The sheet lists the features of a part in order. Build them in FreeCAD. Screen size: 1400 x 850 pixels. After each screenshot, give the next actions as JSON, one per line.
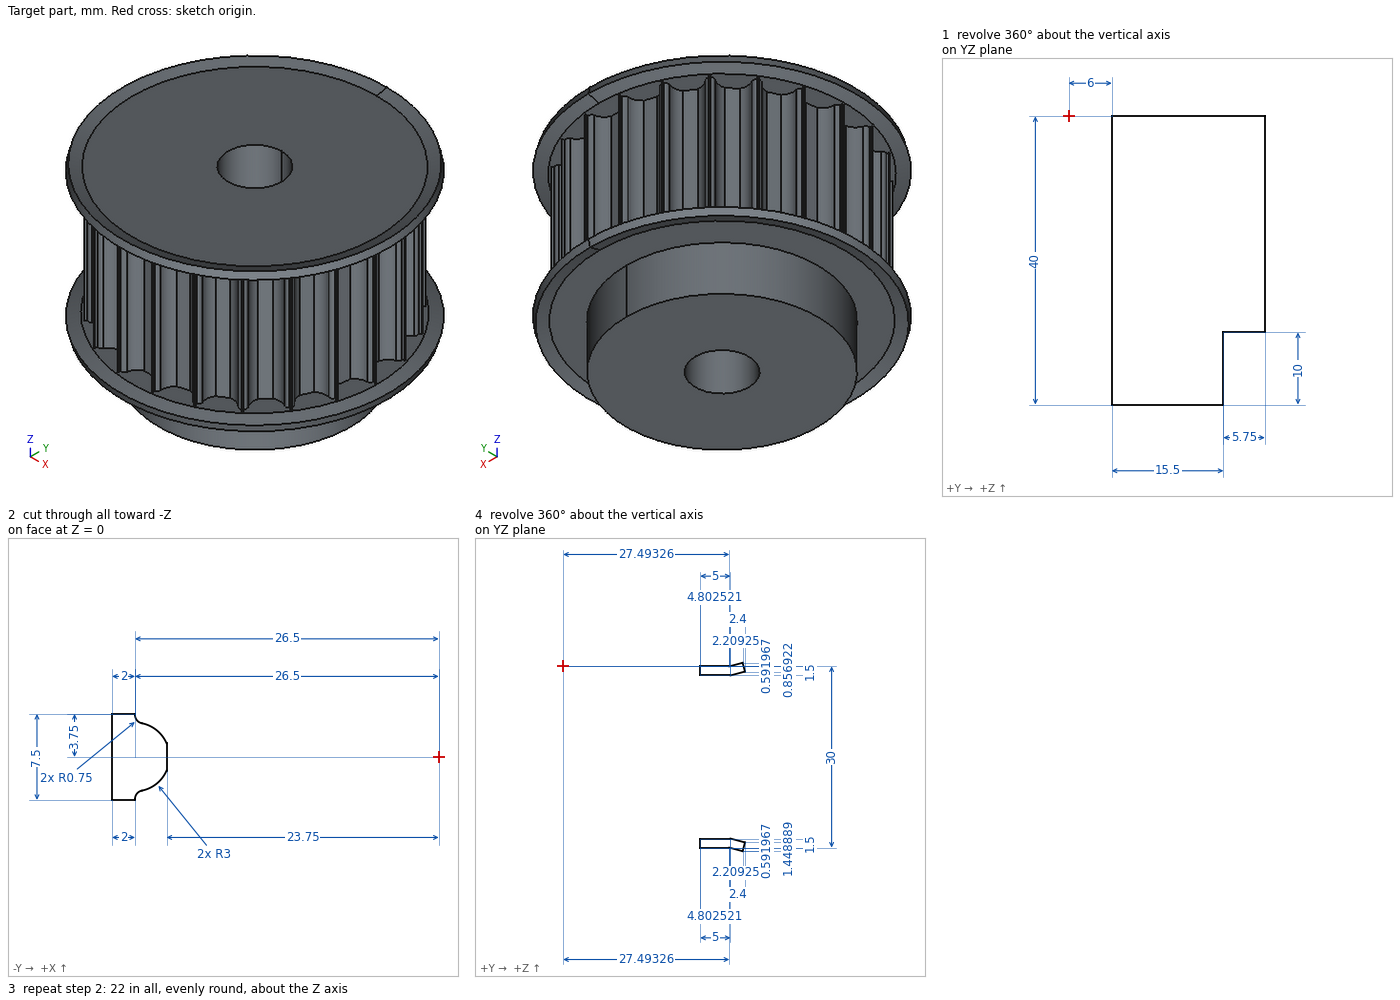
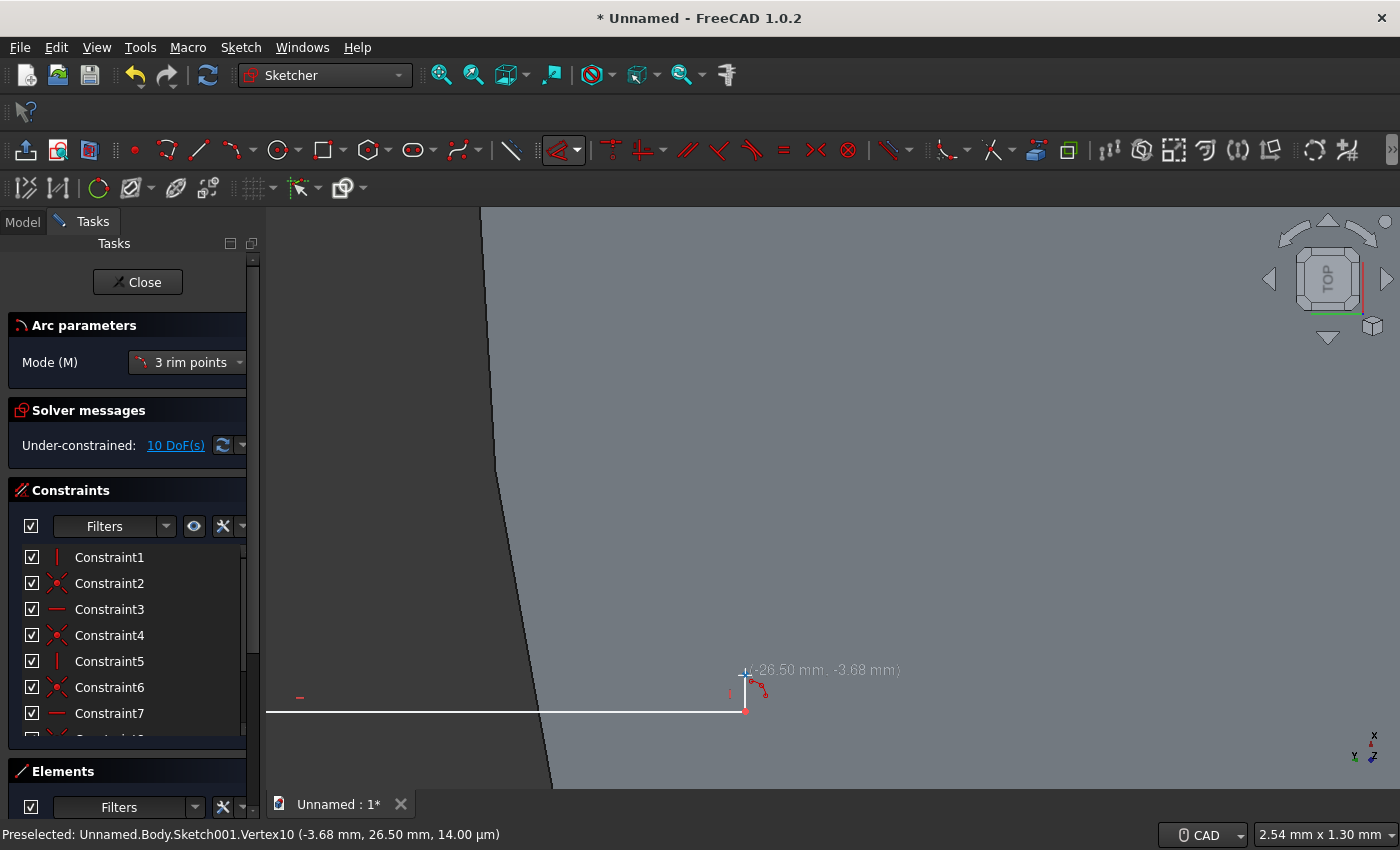
{"action": "scroll", "coordinate": [746, 681], "scroll_direction": "down", "scroll_amount": 11}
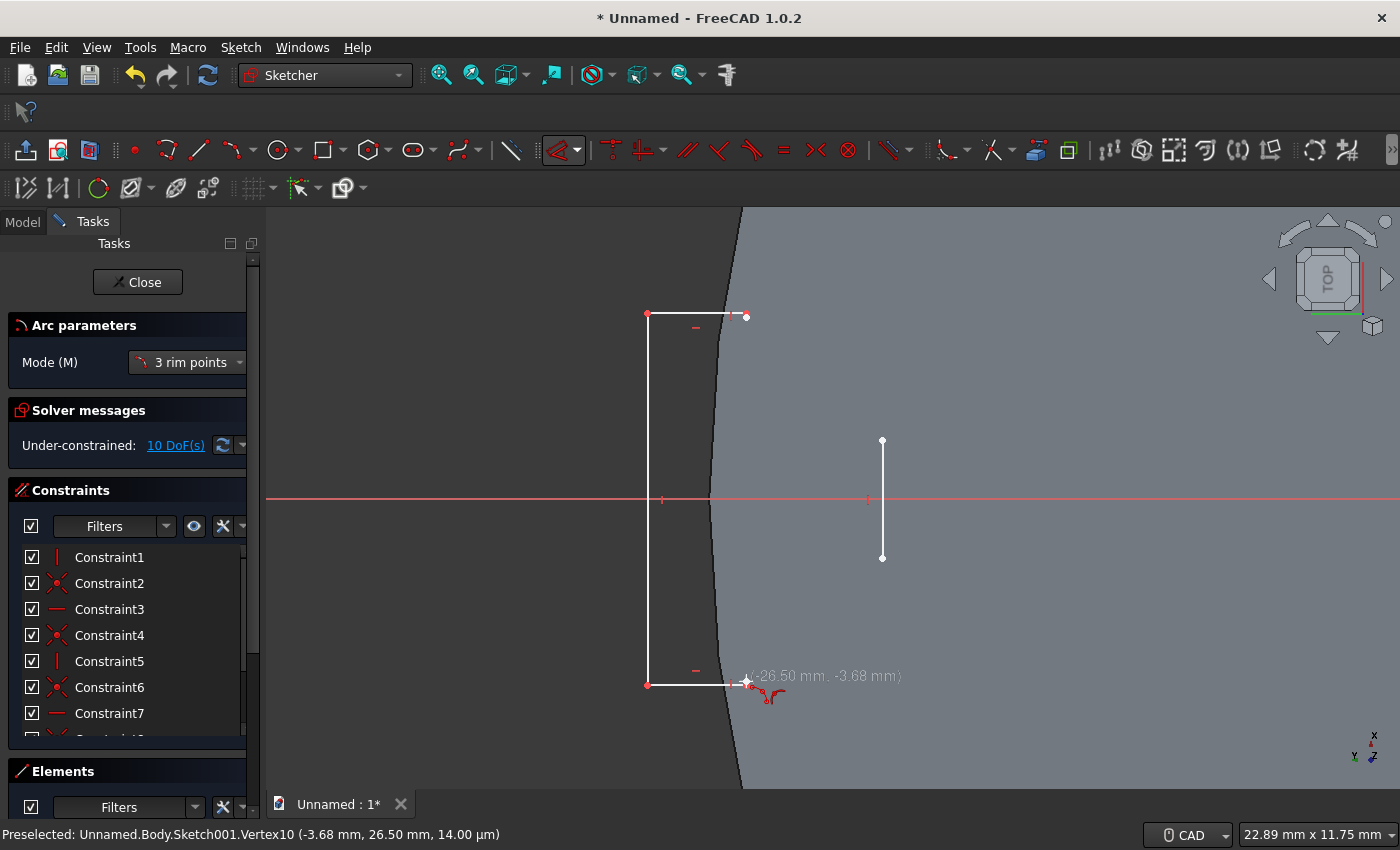
{"action": "left_click", "coordinate": [776, 644]}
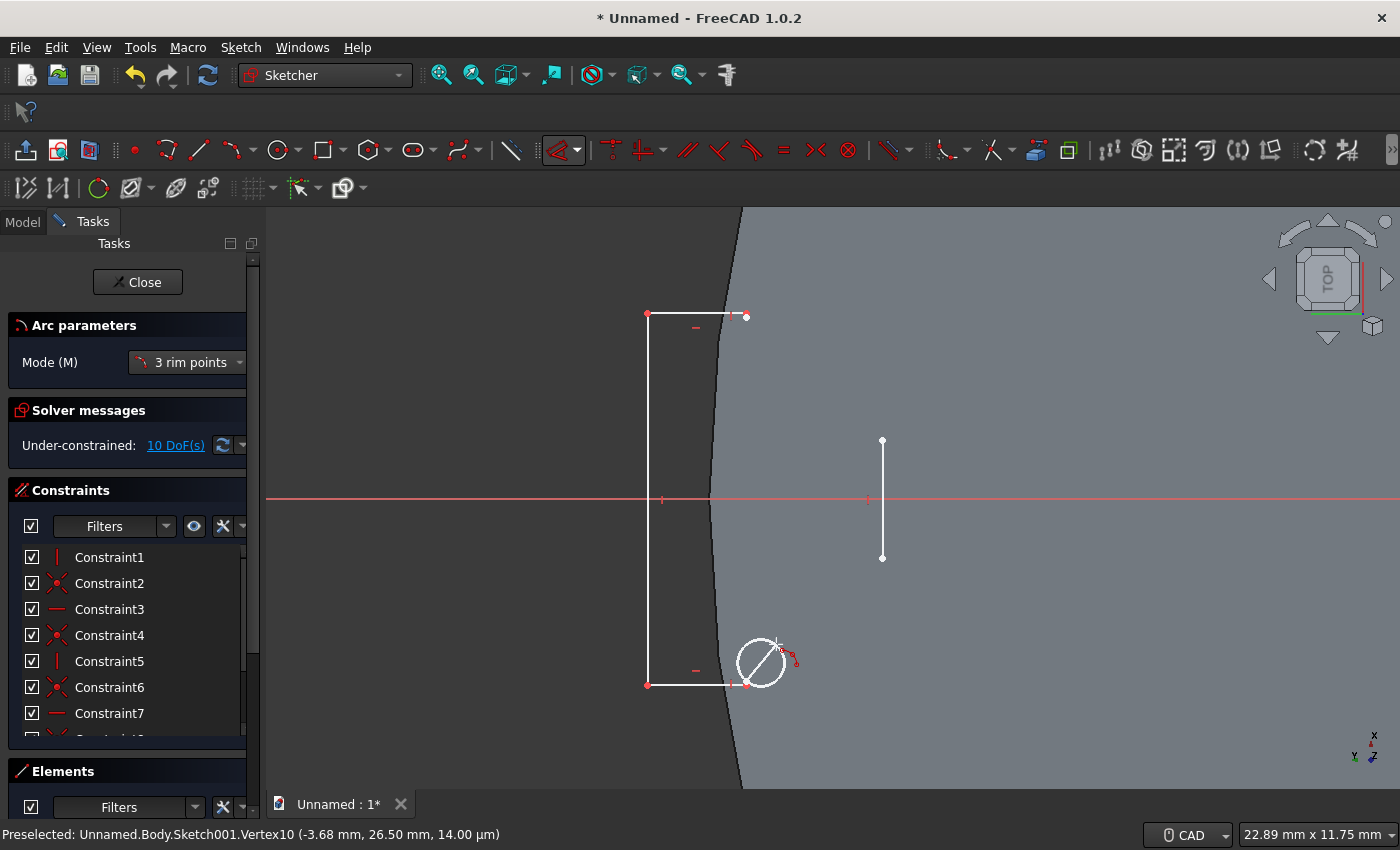
{"action": "scroll", "coordinate": [755, 657], "scroll_direction": "up", "scroll_amount": 4}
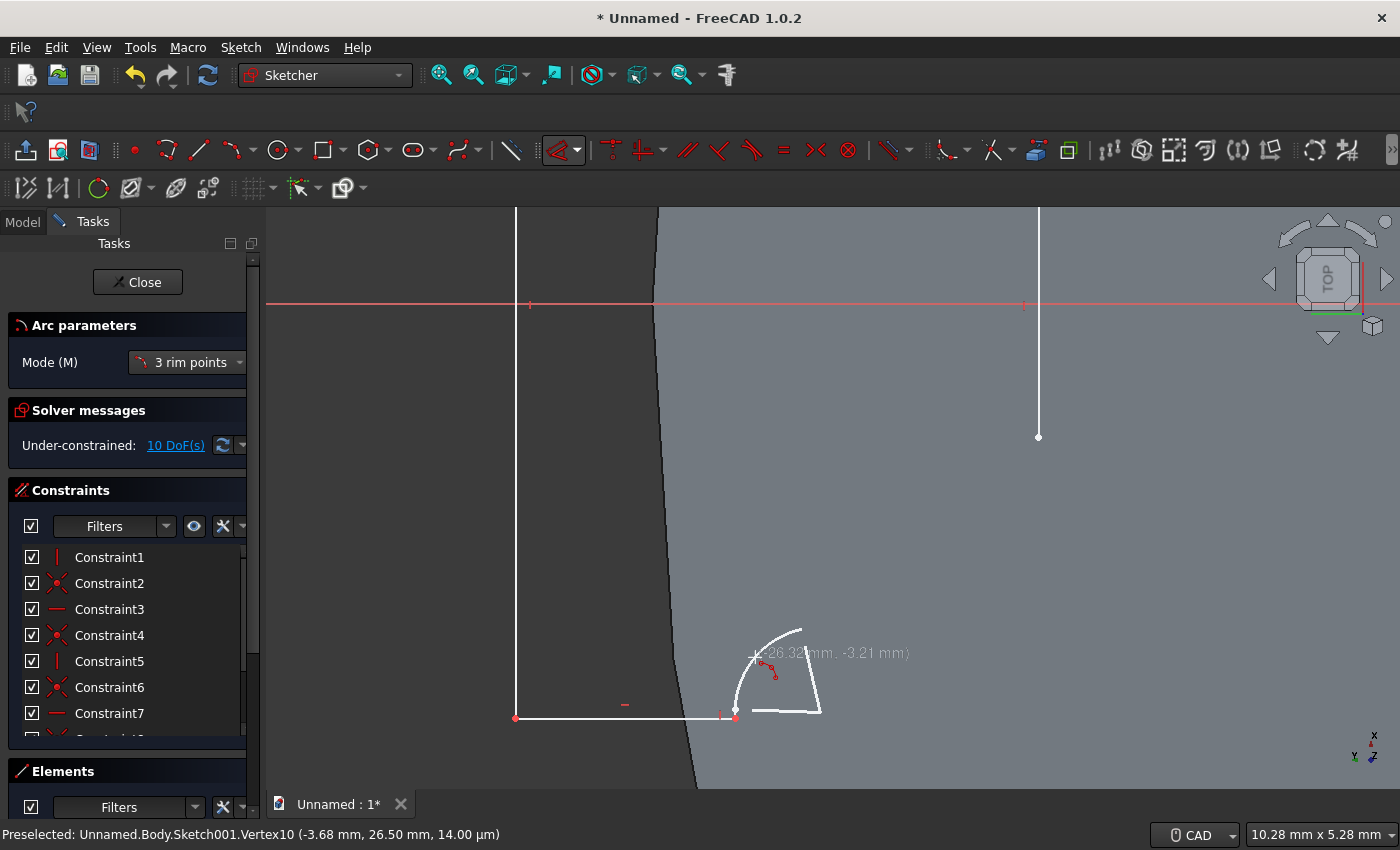
{"action": "left_click", "coordinate": [754, 657]}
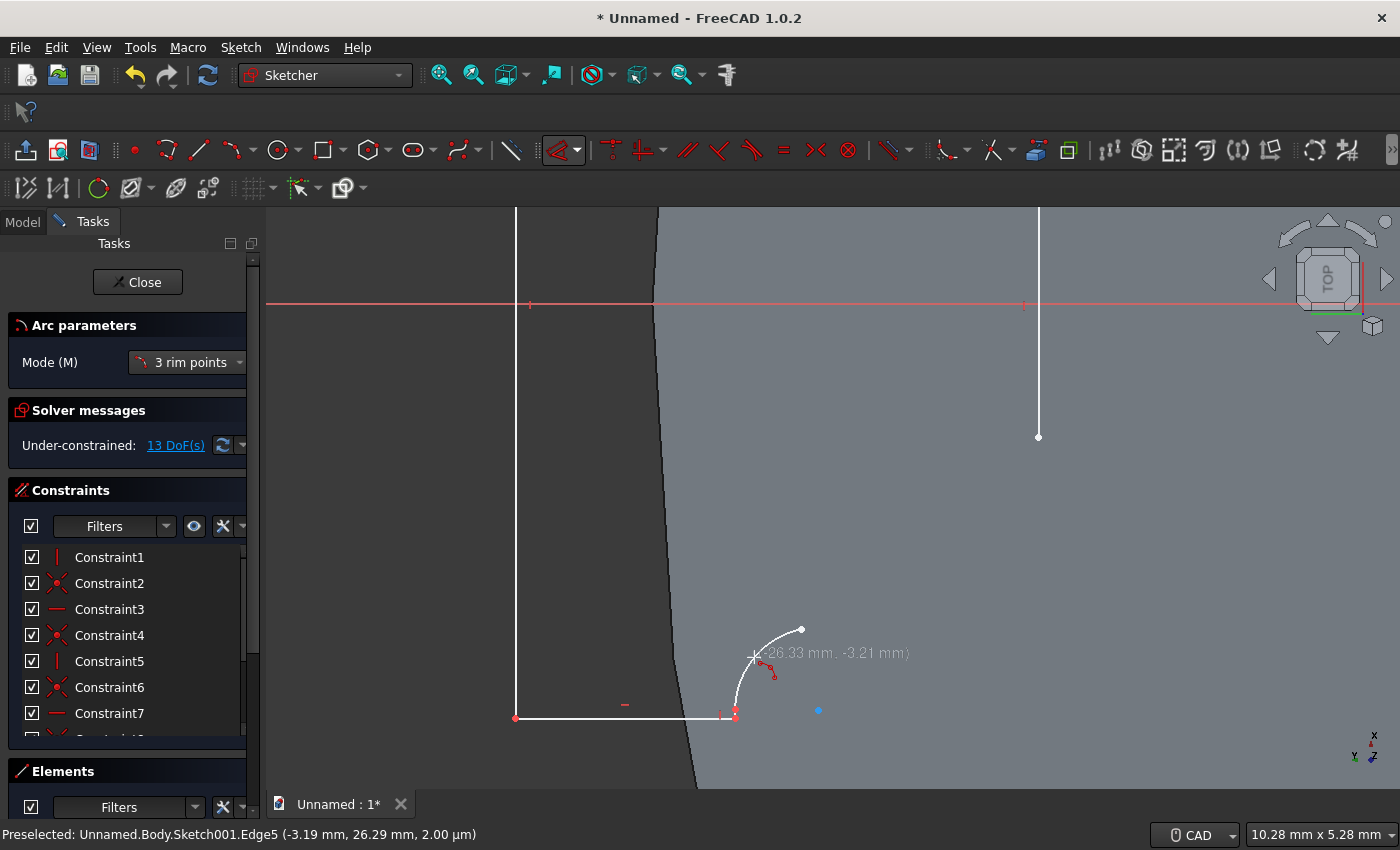
{"action": "left_click", "coordinate": [801, 629]}
{"action": "left_click", "coordinate": [1039, 437]}
{"action": "left_click", "coordinate": [943, 561]}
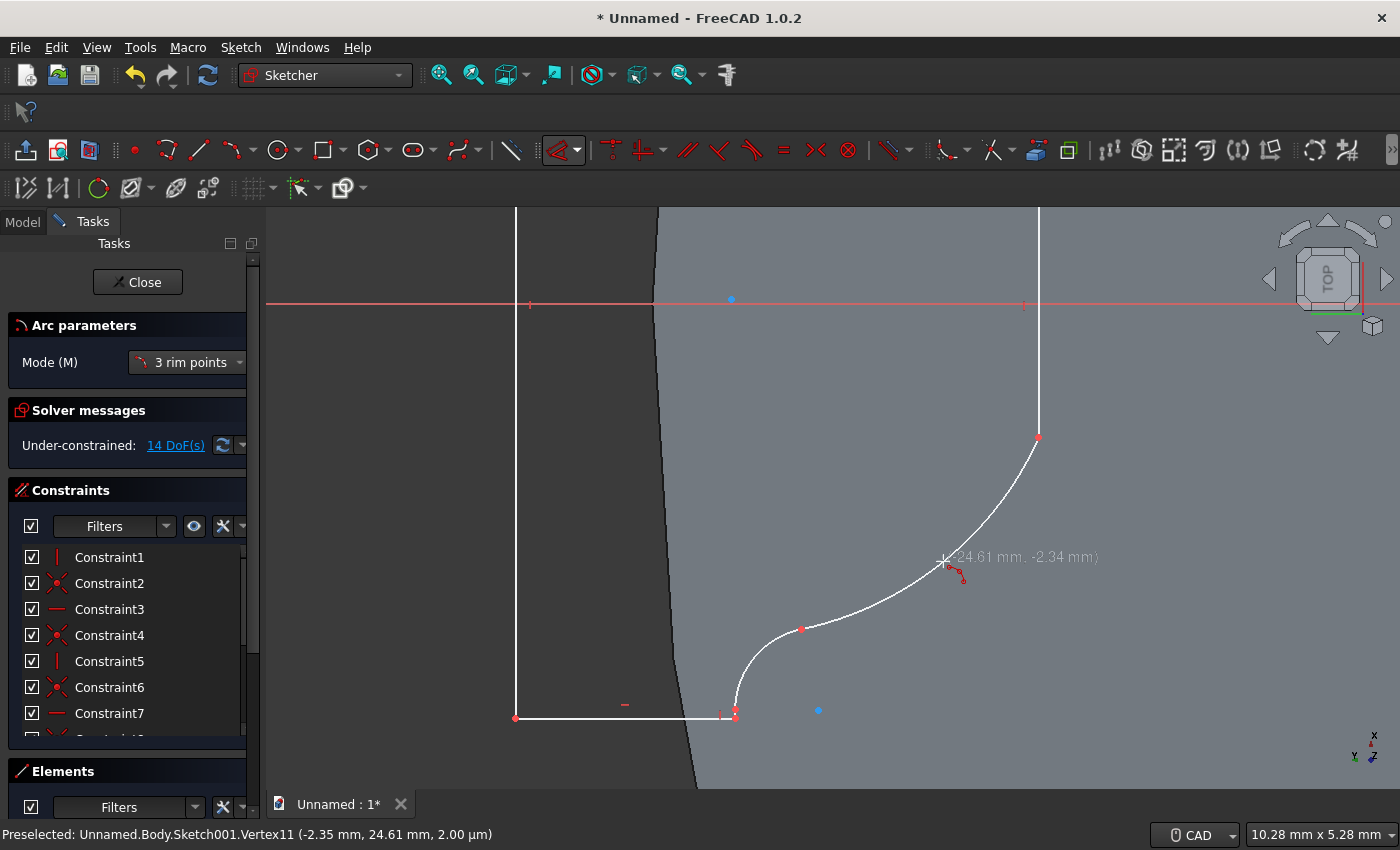
{"action": "scroll", "coordinate": [755, 656], "scroll_direction": "down", "scroll_amount": 4}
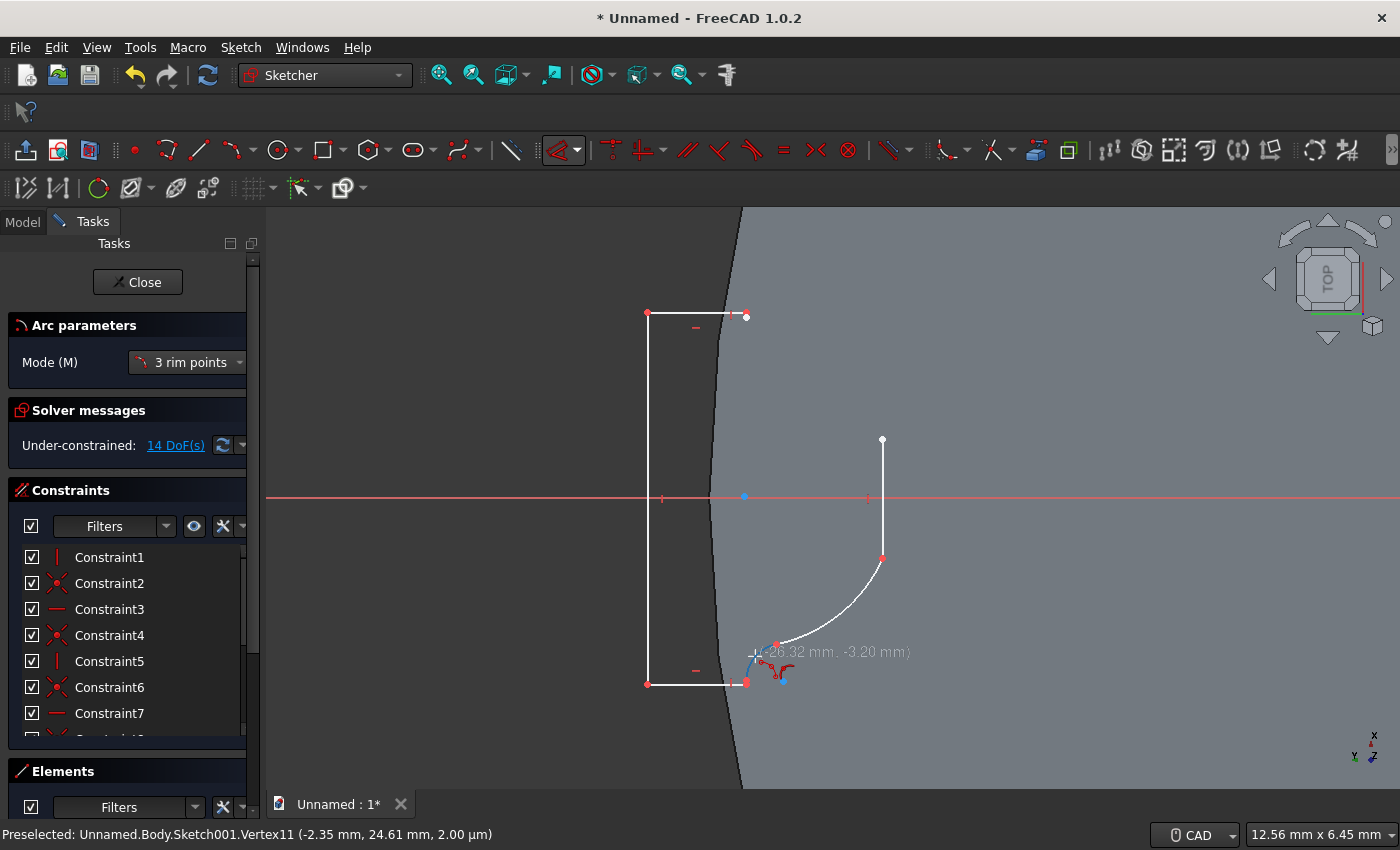
{"action": "left_click", "coordinate": [883, 440]}
{"action": "left_click", "coordinate": [776, 353]}
{"action": "left_click", "coordinate": [840, 383]}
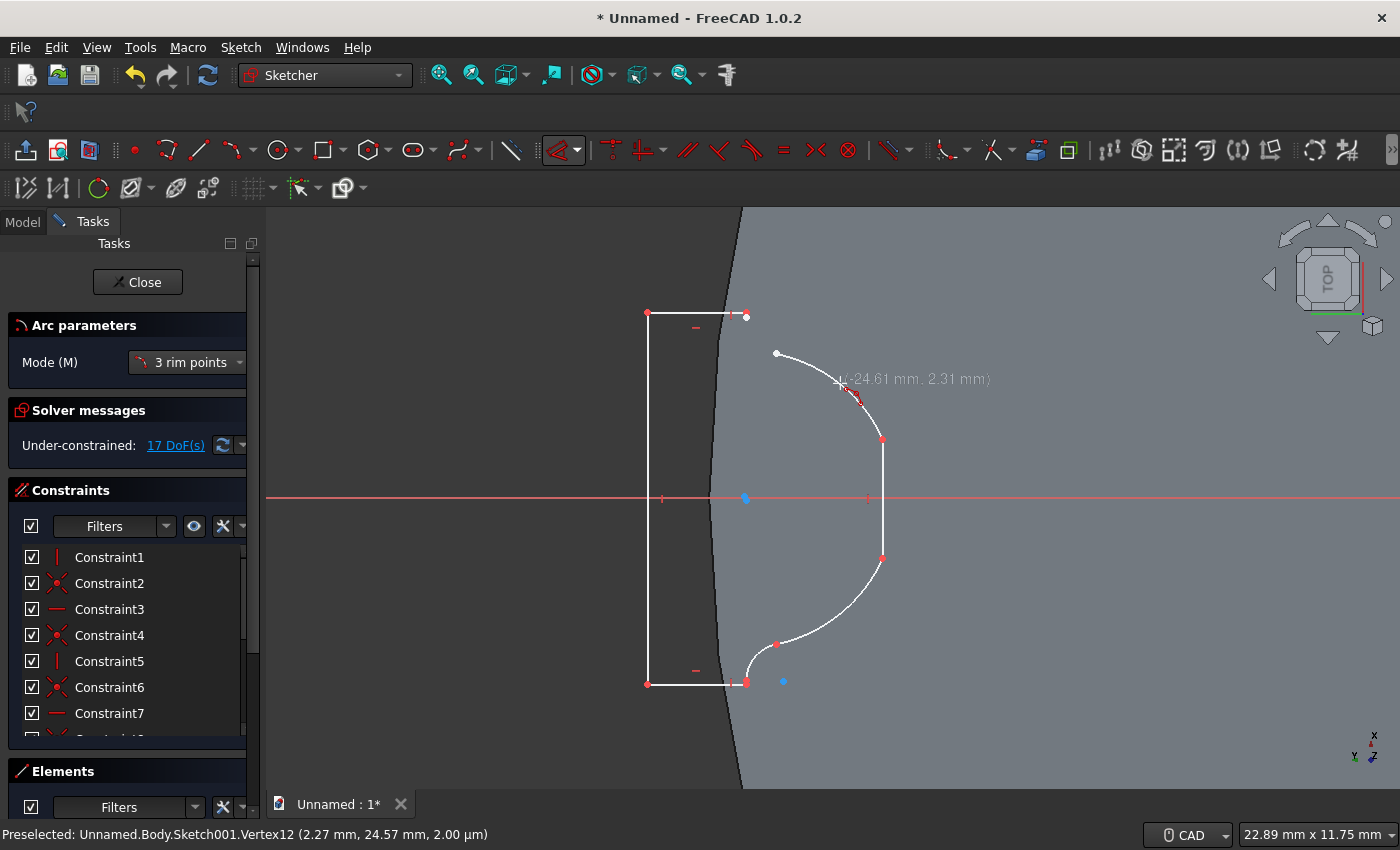
{"action": "left_click", "coordinate": [776, 354]}